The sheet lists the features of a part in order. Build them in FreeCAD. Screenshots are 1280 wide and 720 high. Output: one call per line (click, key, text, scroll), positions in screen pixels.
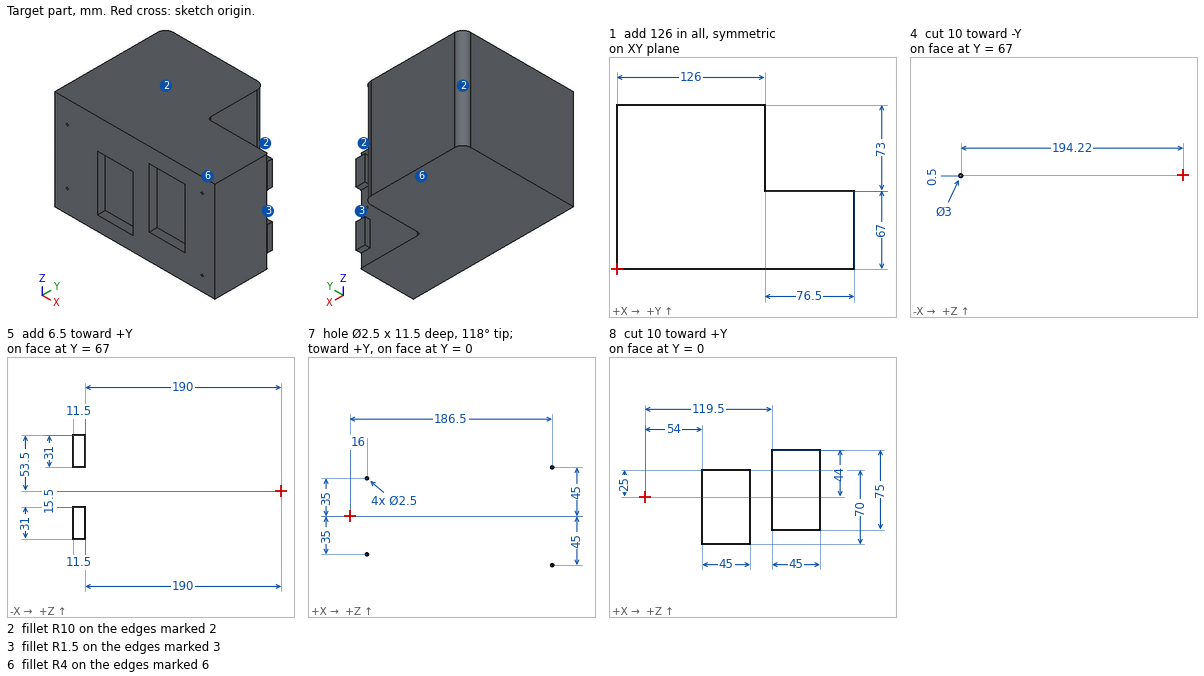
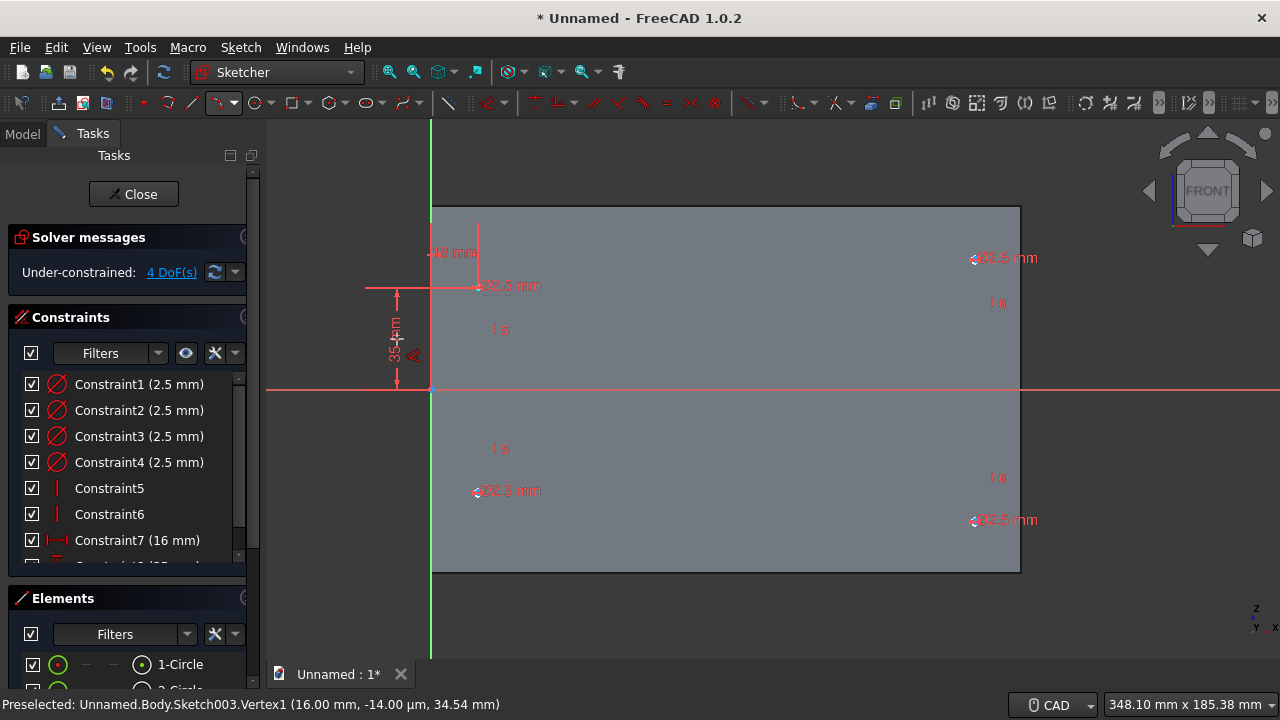
click(478, 493)
click(397, 441)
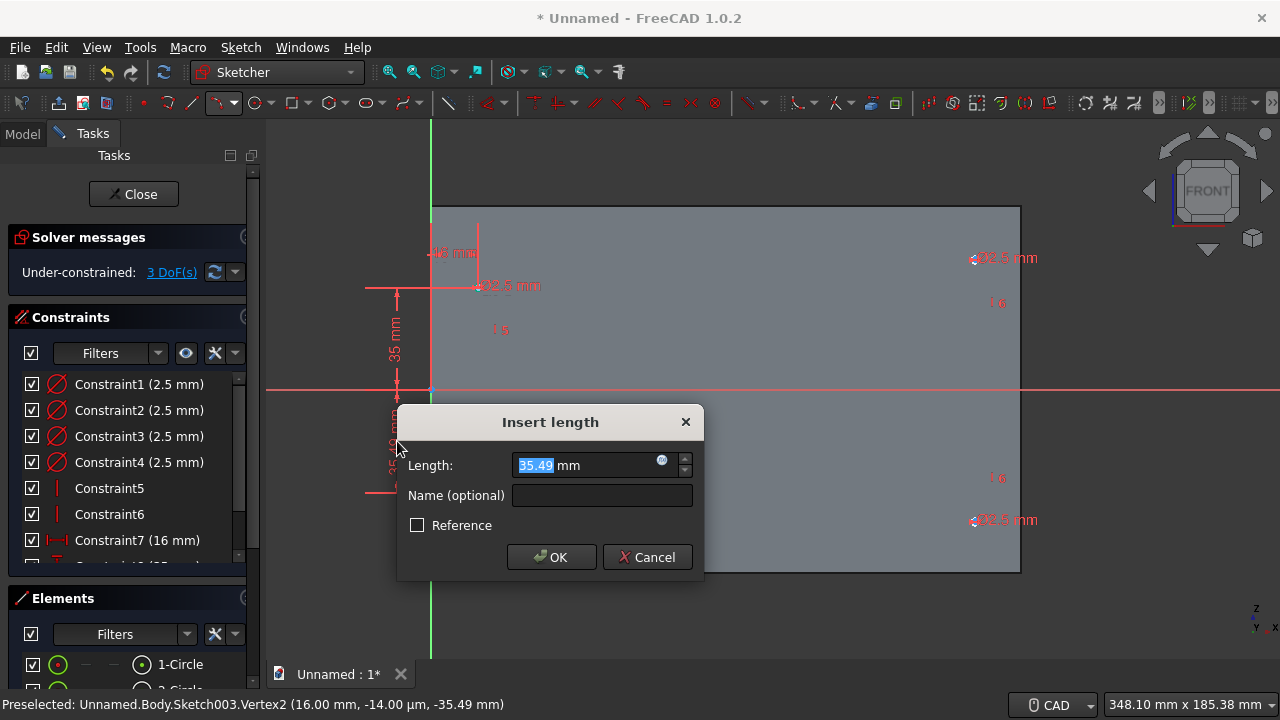
text(35)
key(Return)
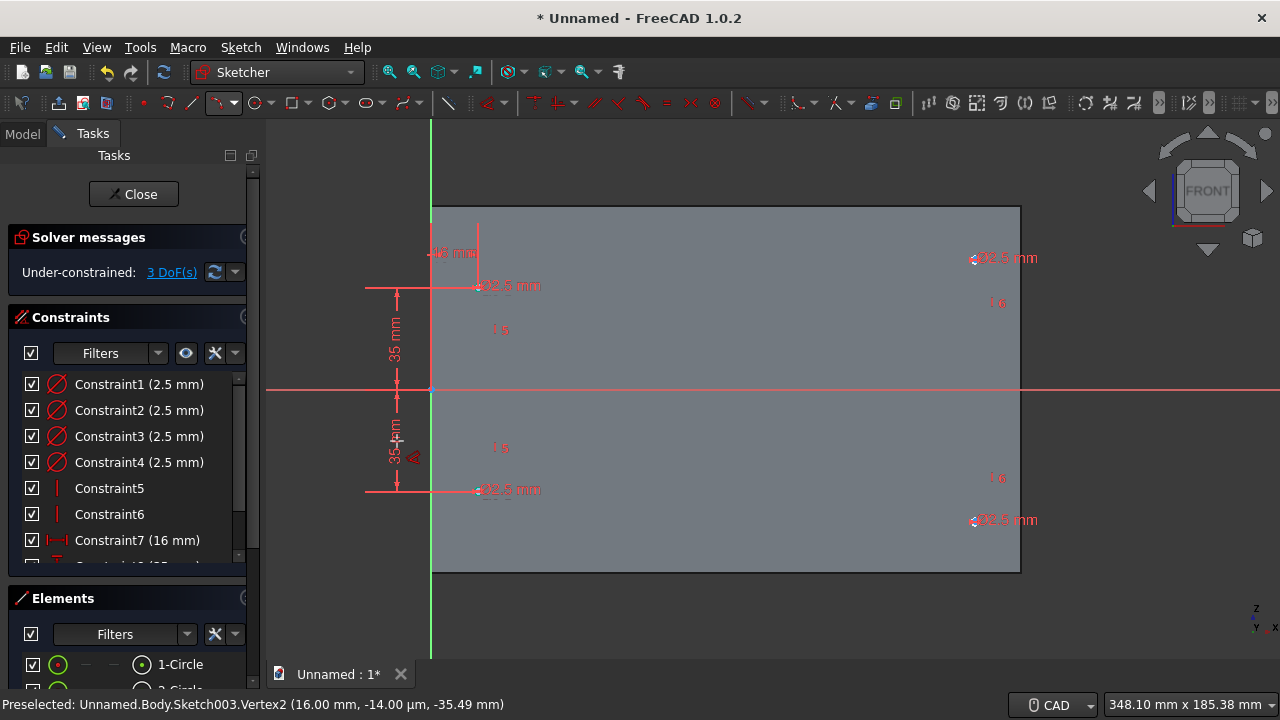
click(975, 260)
click(397, 295)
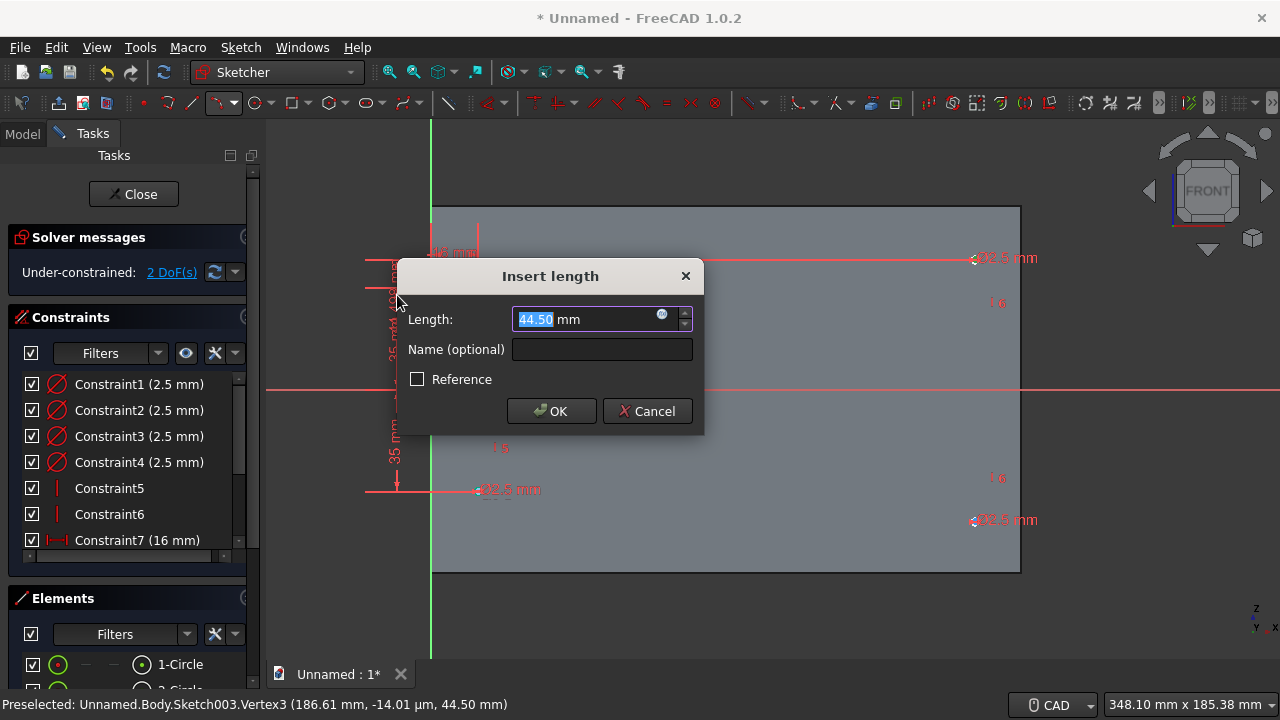
text(45)
key(Return)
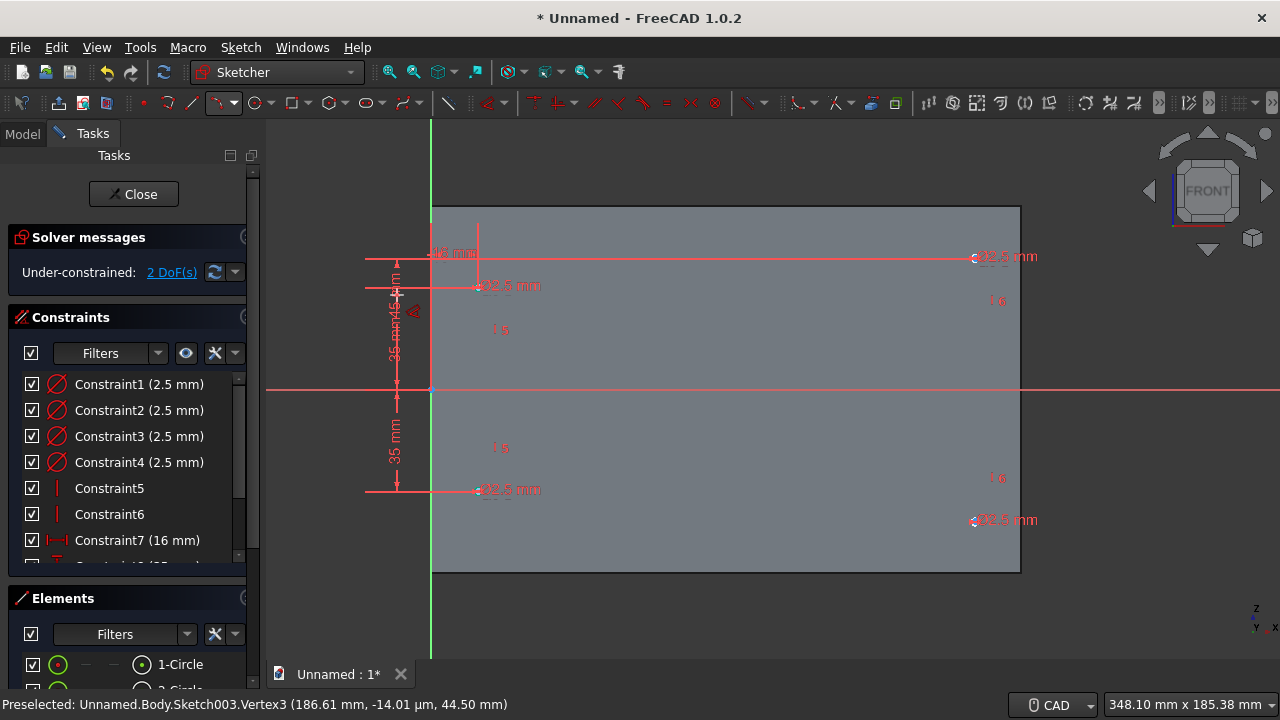
click(975, 522)
click(397, 486)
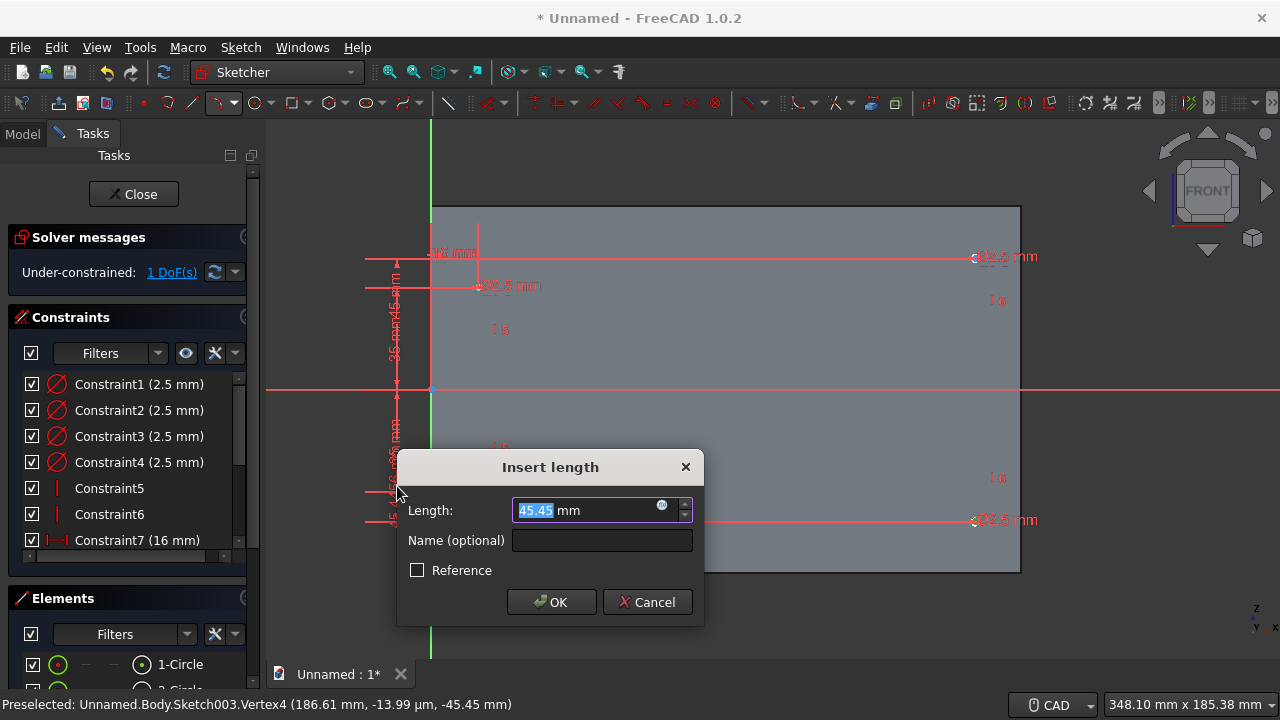
text(45)
key(Return)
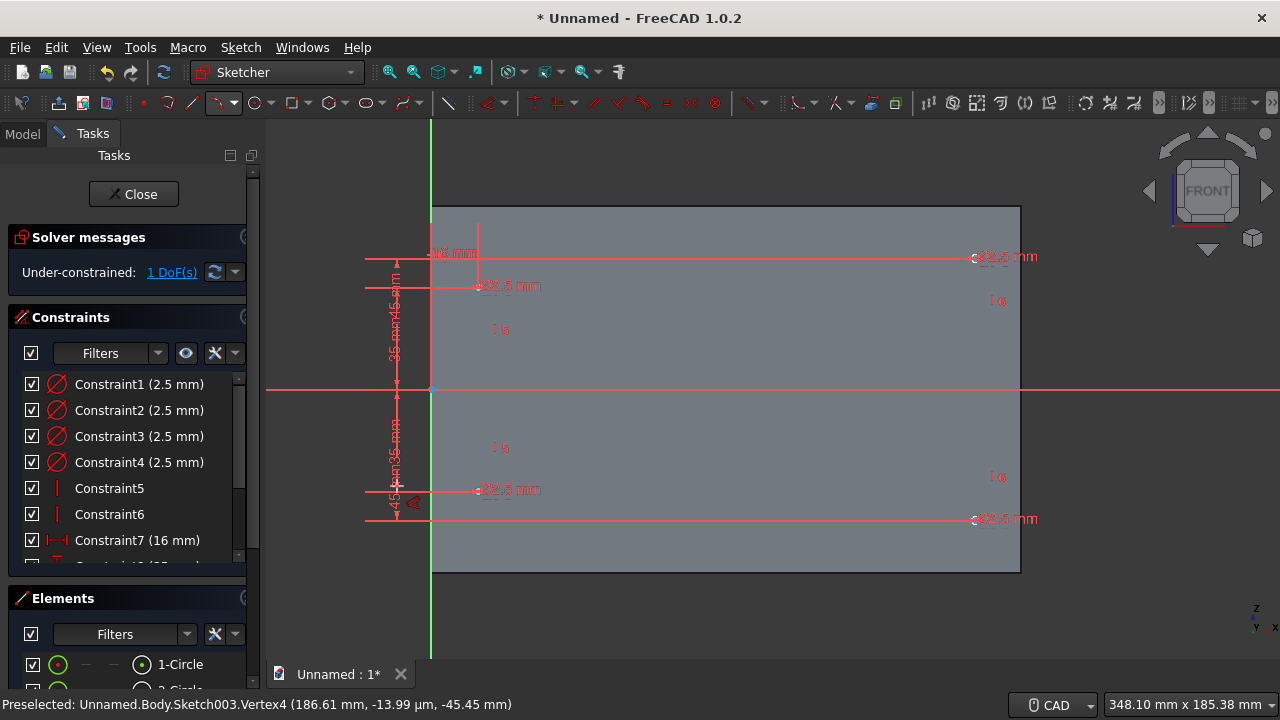
click(975, 259)
click(703, 225)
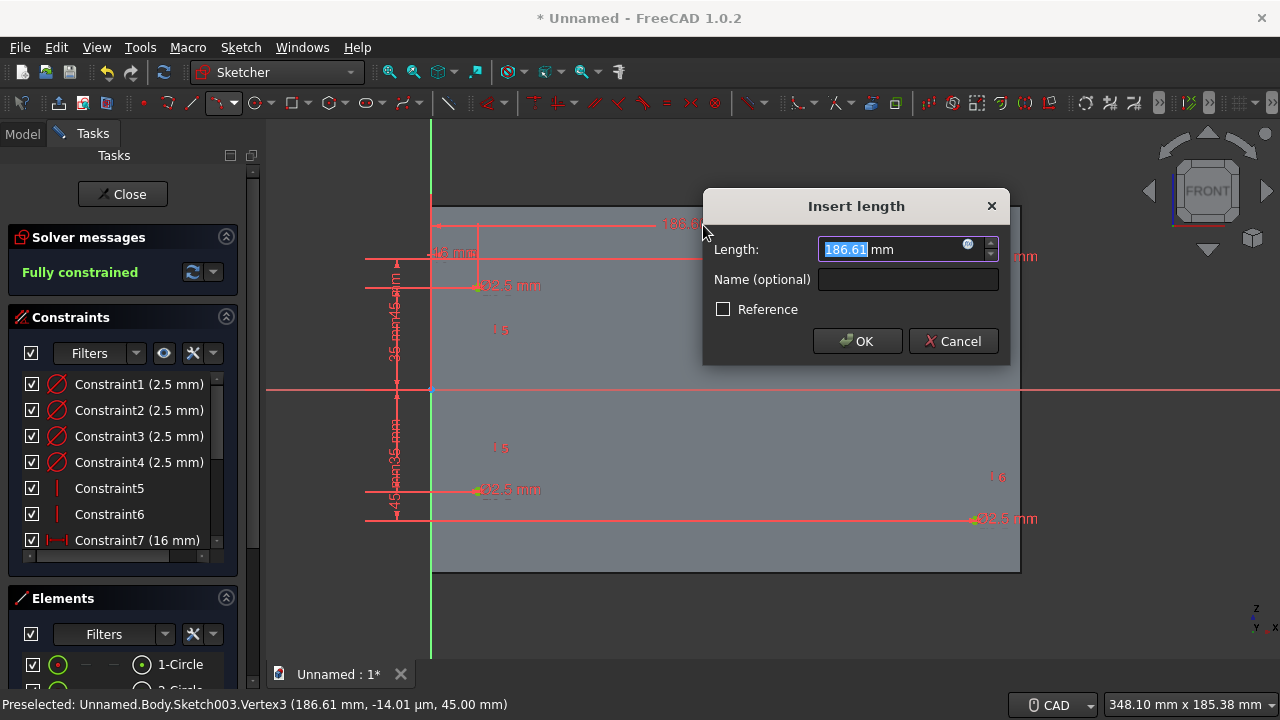
text(186.5)
key(Return)
key(Escape)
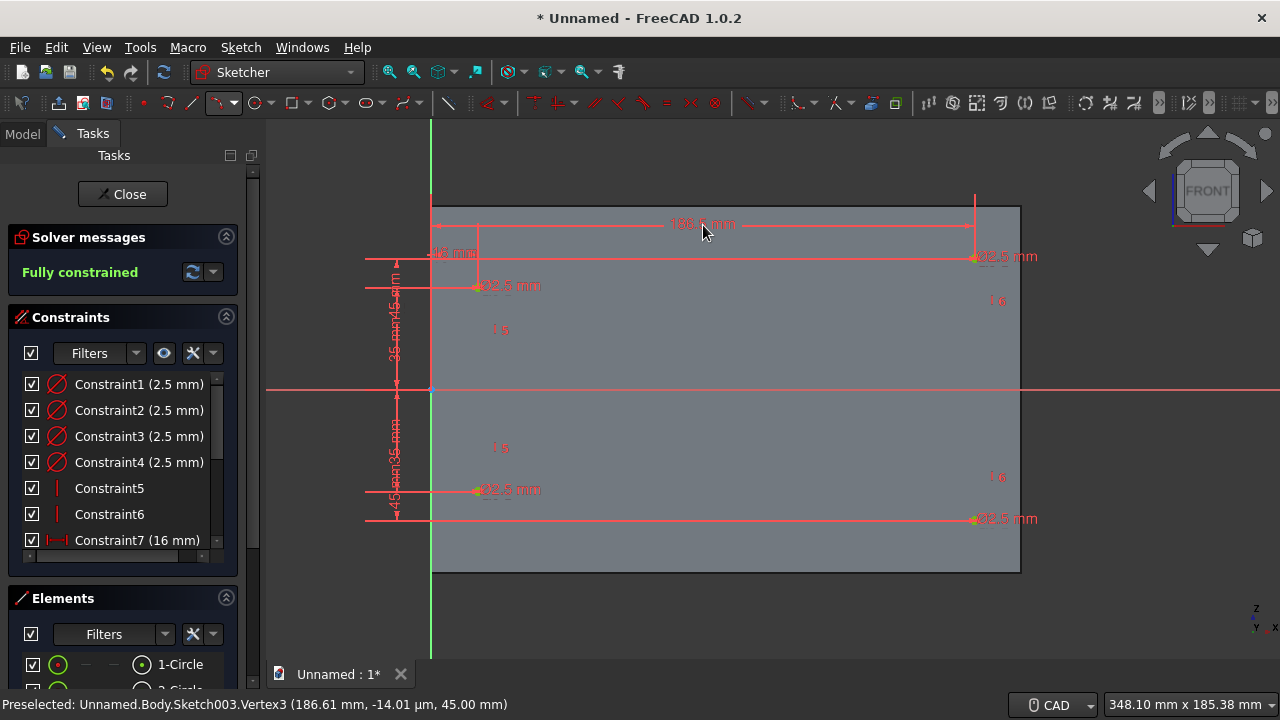
click(123, 194)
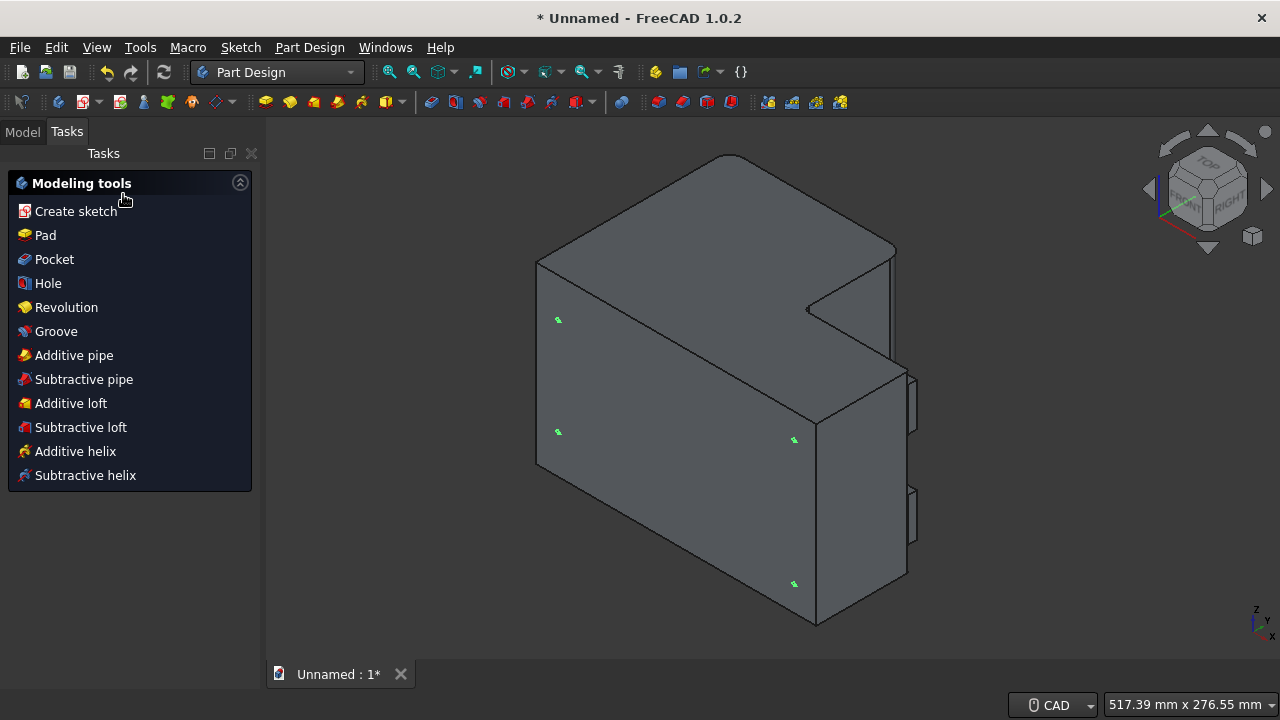
click(456, 102)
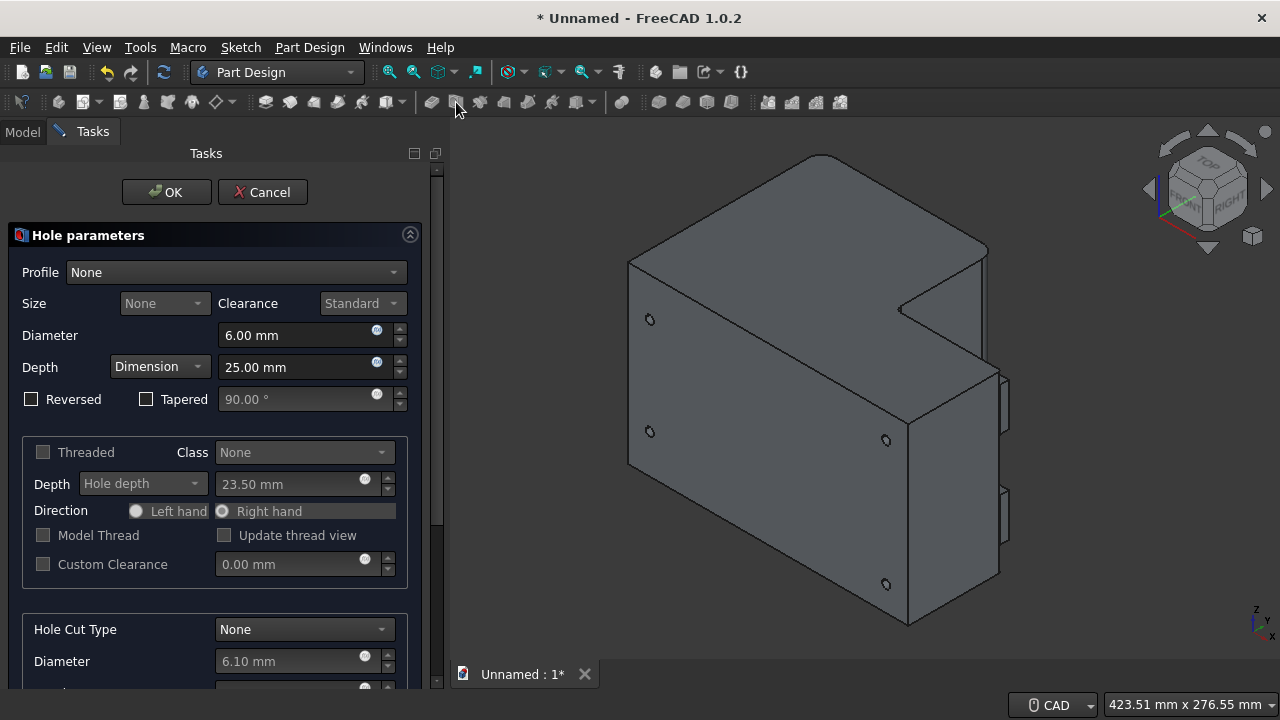
triple_click(305, 335)